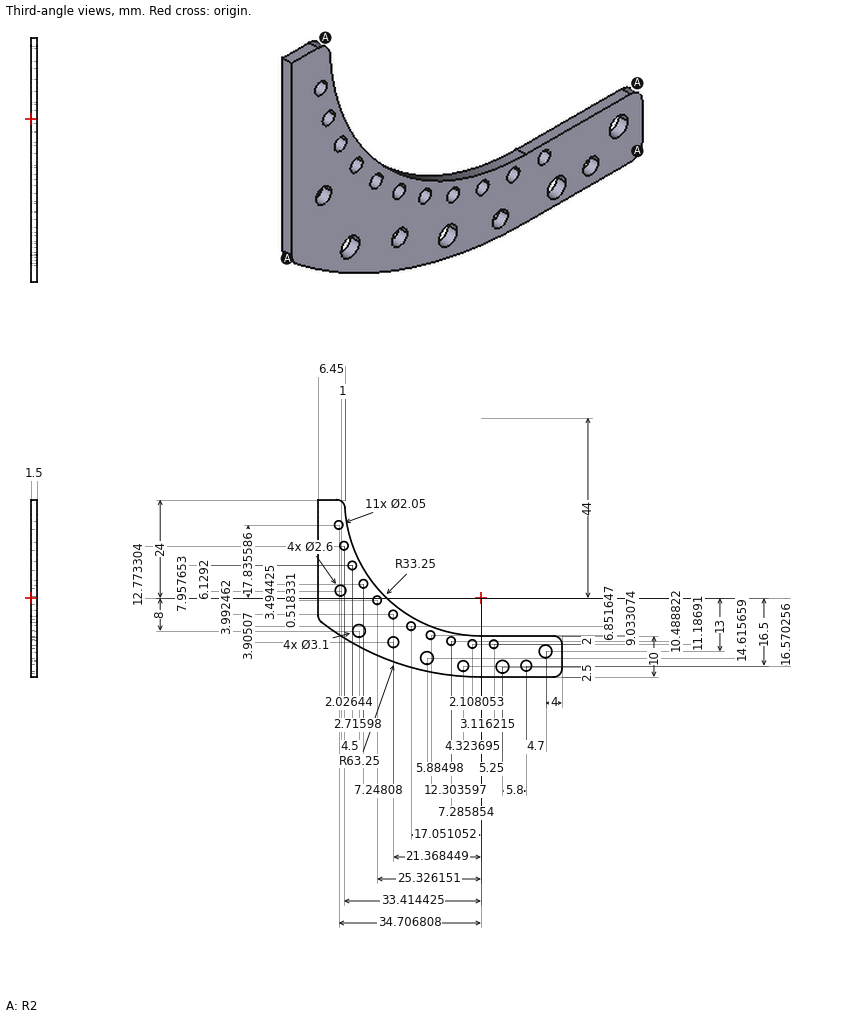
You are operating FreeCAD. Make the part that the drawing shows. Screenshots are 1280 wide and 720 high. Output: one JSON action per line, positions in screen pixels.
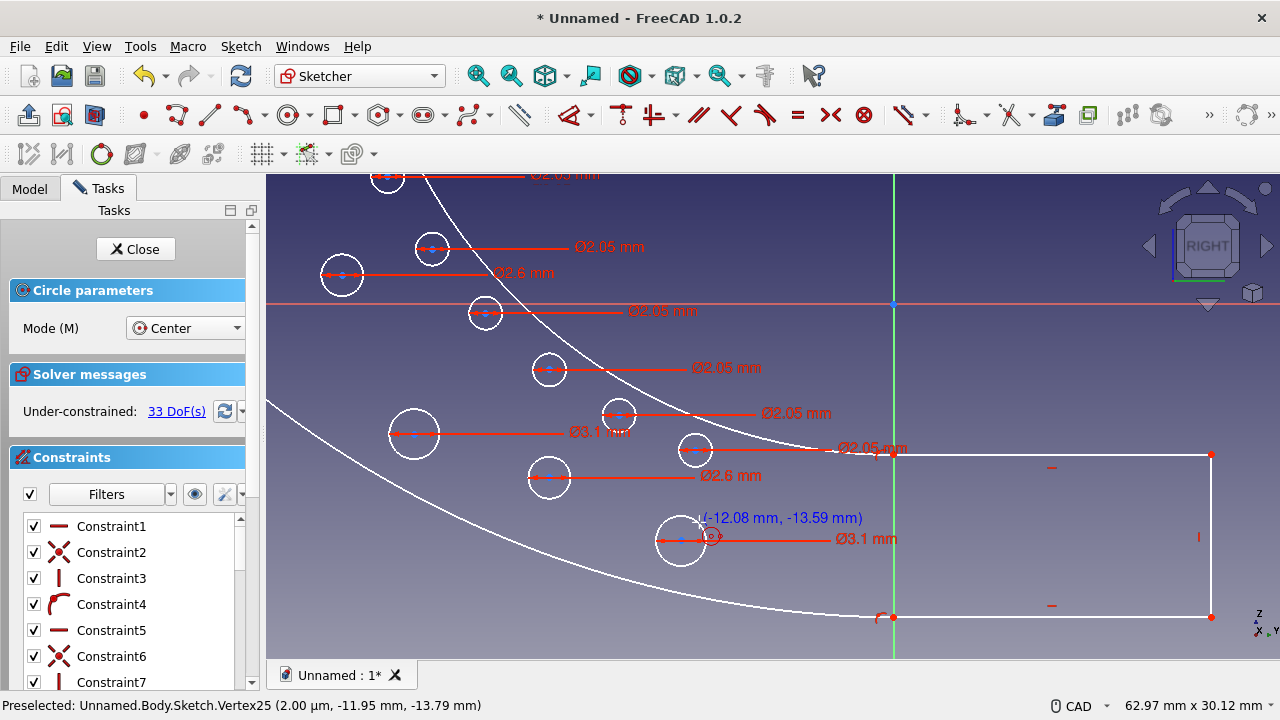
{"action": "scroll", "coordinate": [776, 473], "scroll_direction": "up", "scroll_amount": 2}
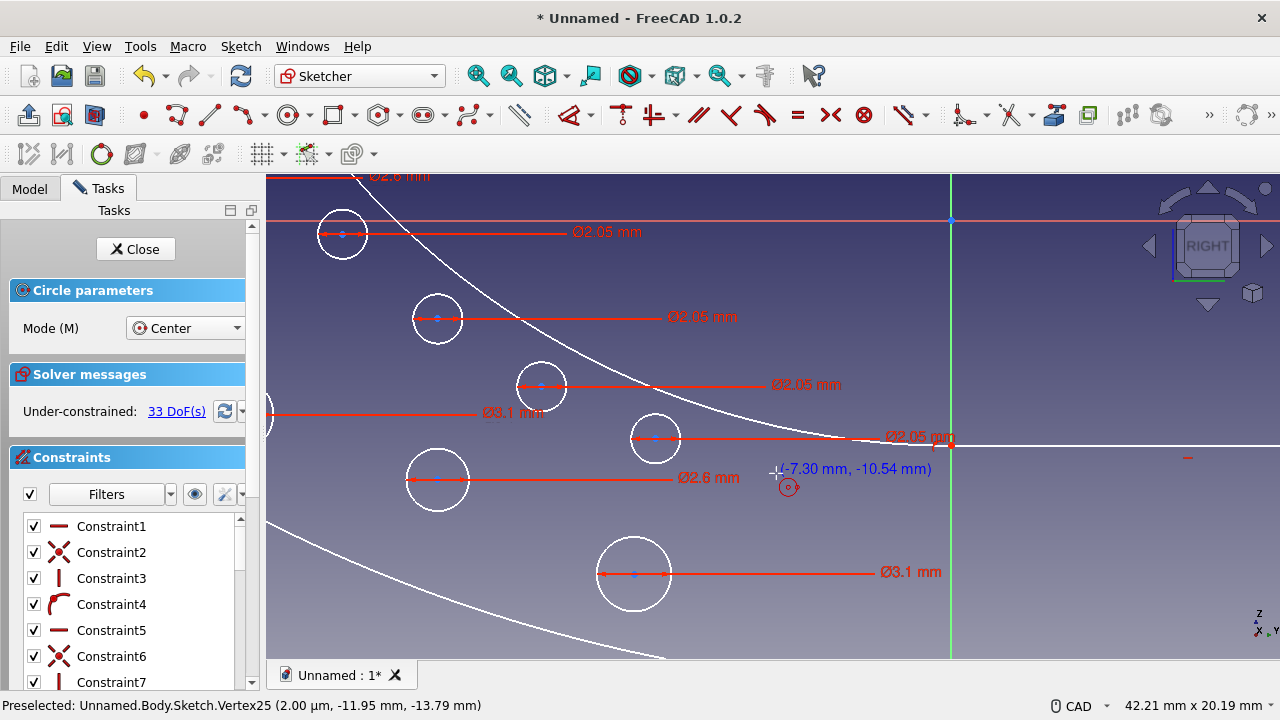
{"action": "left_click", "coordinate": [776, 473]}
{"action": "mouse_move", "coordinate": [794, 455]}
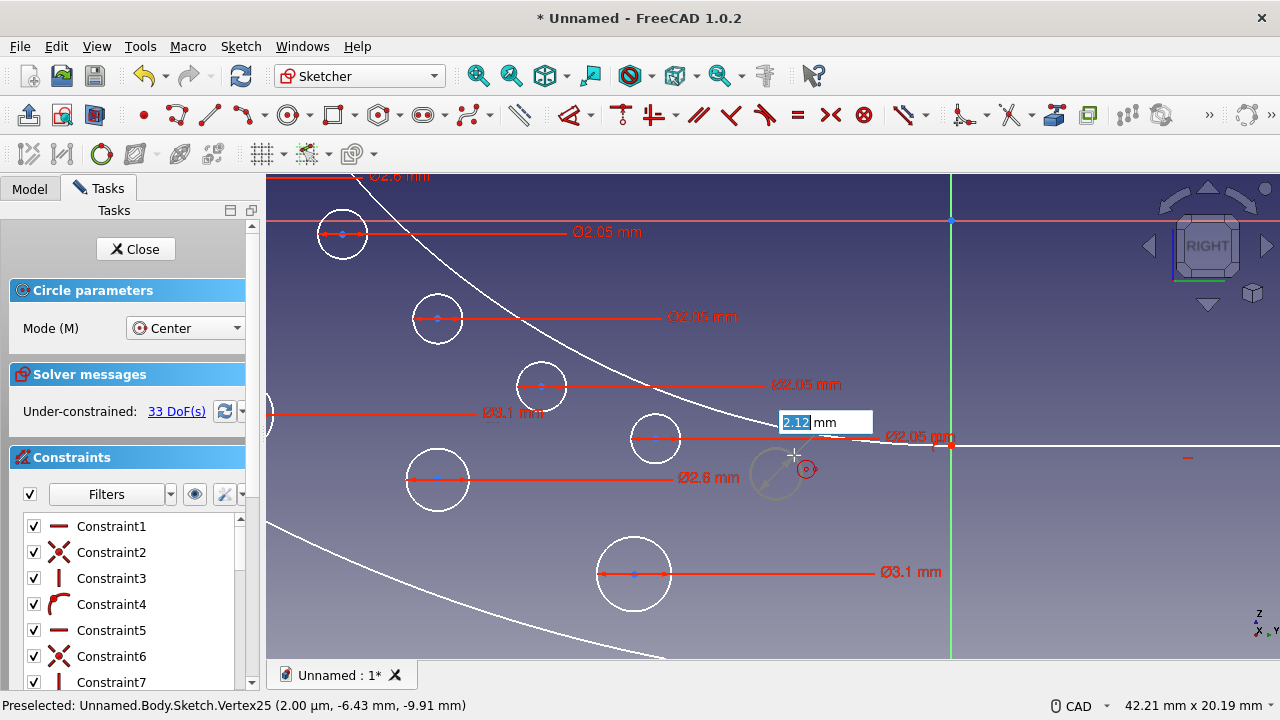
{"action": "type", "text": "2.05"}
{"action": "key", "text": "Return"}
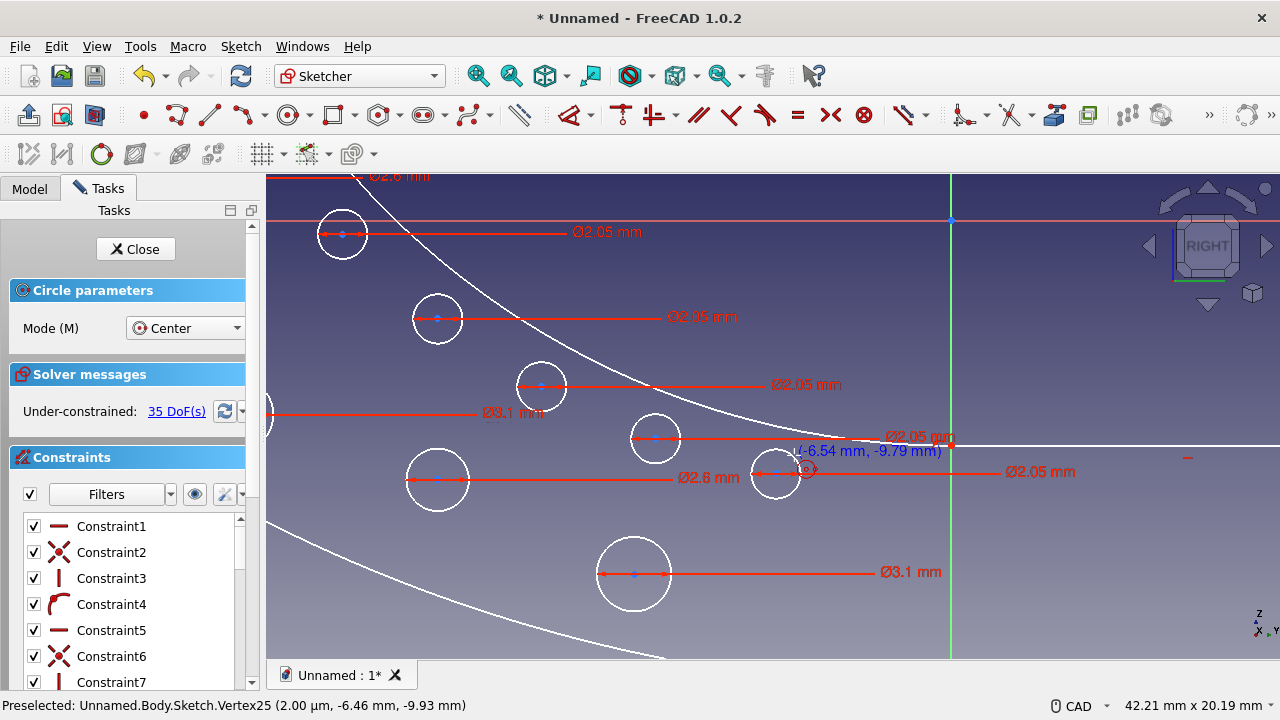
{"action": "left_click", "coordinate": [847, 619]}
{"action": "mouse_move", "coordinate": [869, 597]}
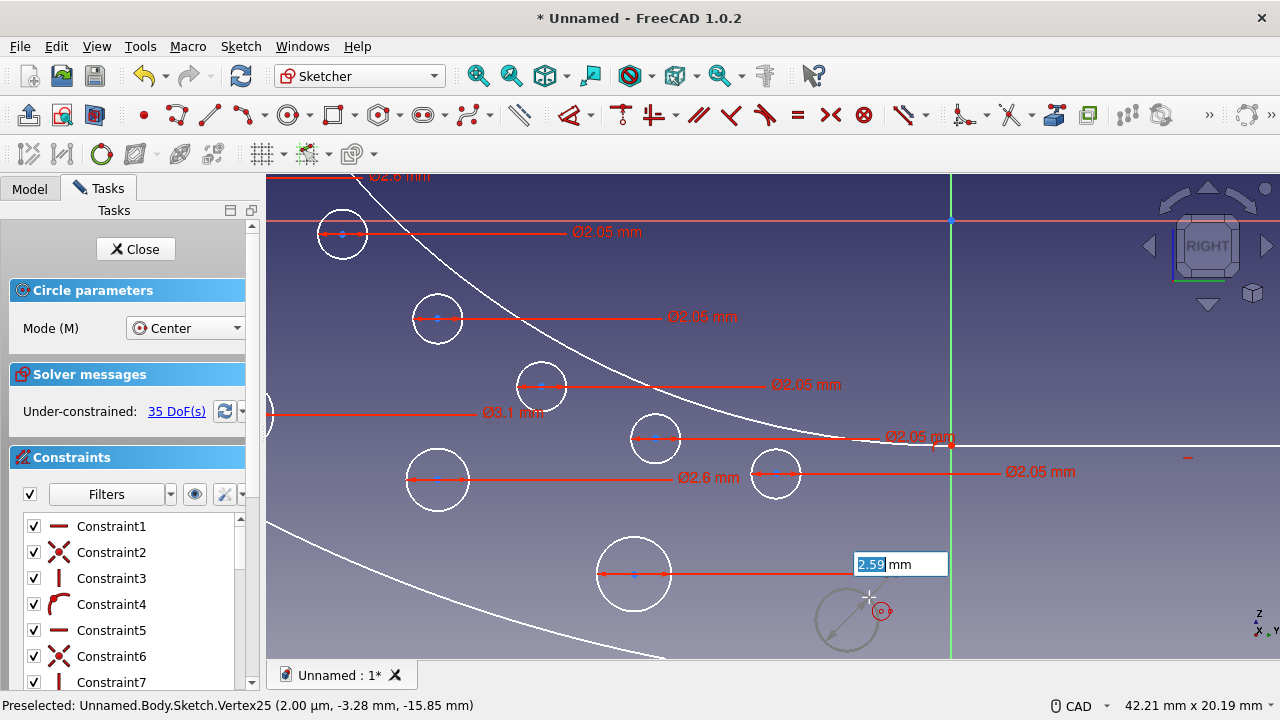
{"action": "type", "text": "2.6"}
{"action": "key", "text": "Return"}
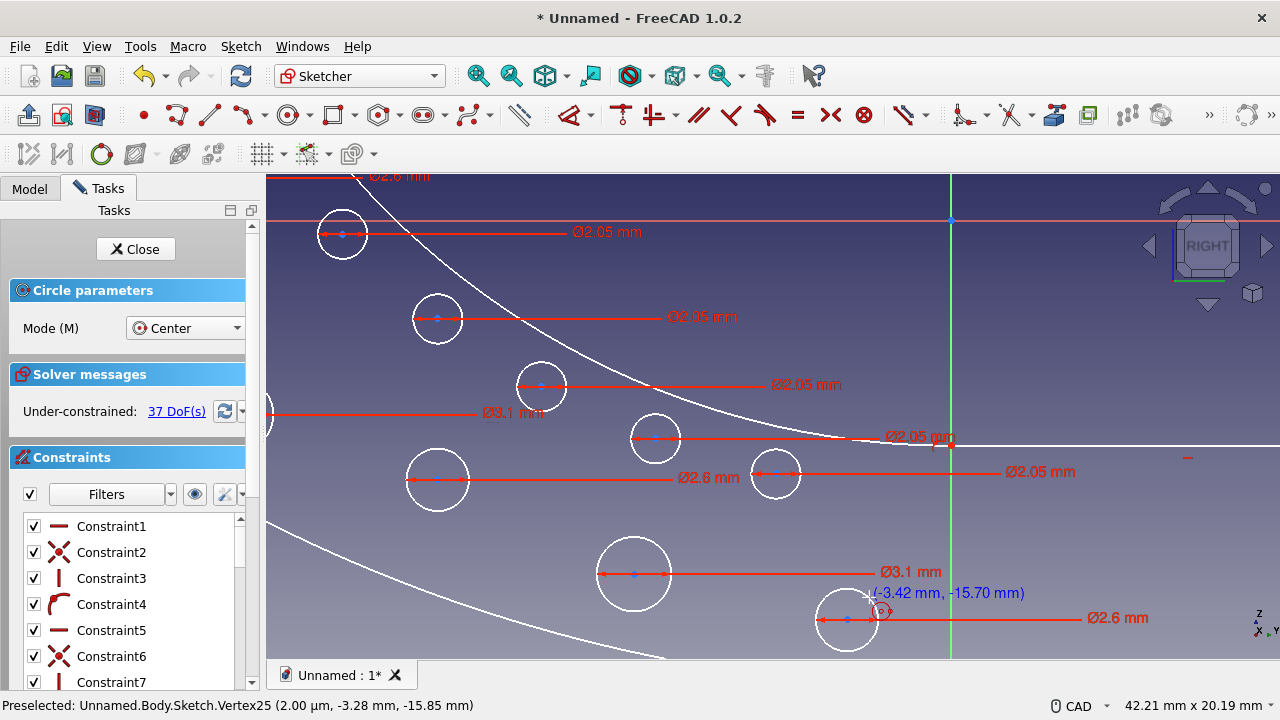
{"action": "left_click", "coordinate": [900, 490]}
{"action": "mouse_move", "coordinate": [918, 472]}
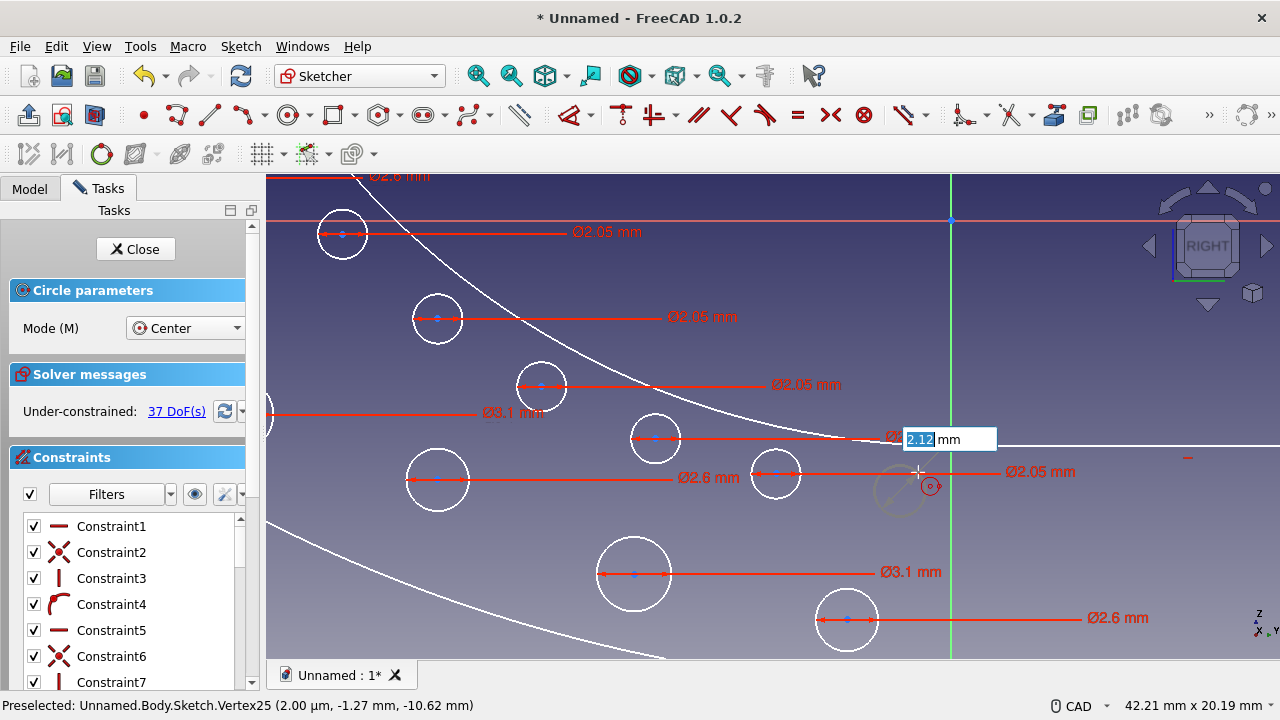
{"action": "type", "text": "2.05"}
{"action": "key", "text": "Return"}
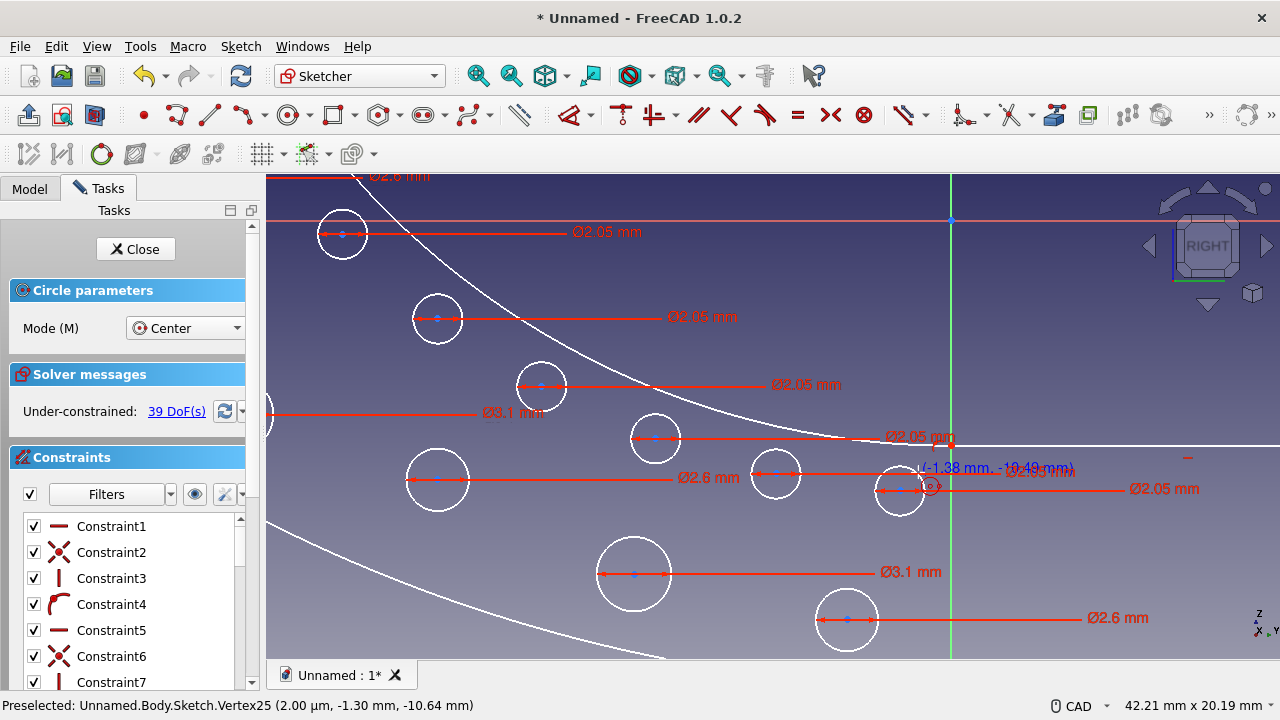
{"action": "left_click", "coordinate": [1026, 491]}
{"action": "mouse_move", "coordinate": [1043, 474]}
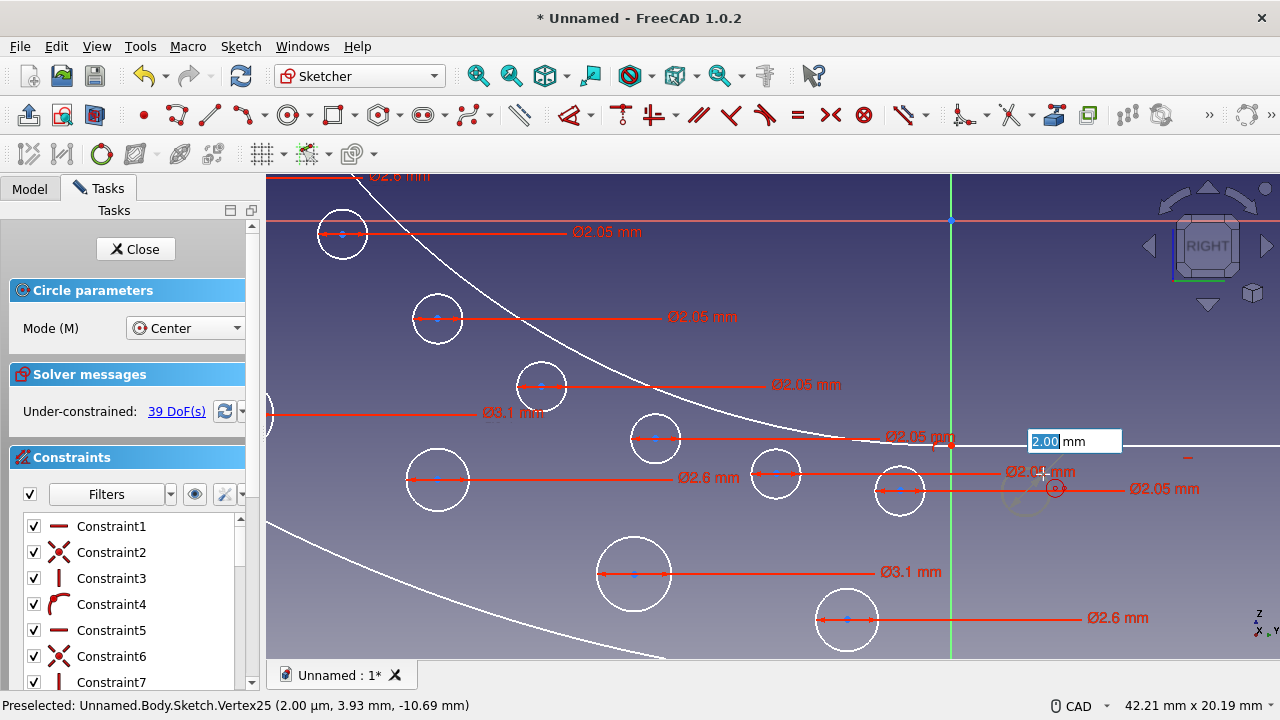
{"action": "type", "text": "2.05"}
{"action": "key", "text": "Return"}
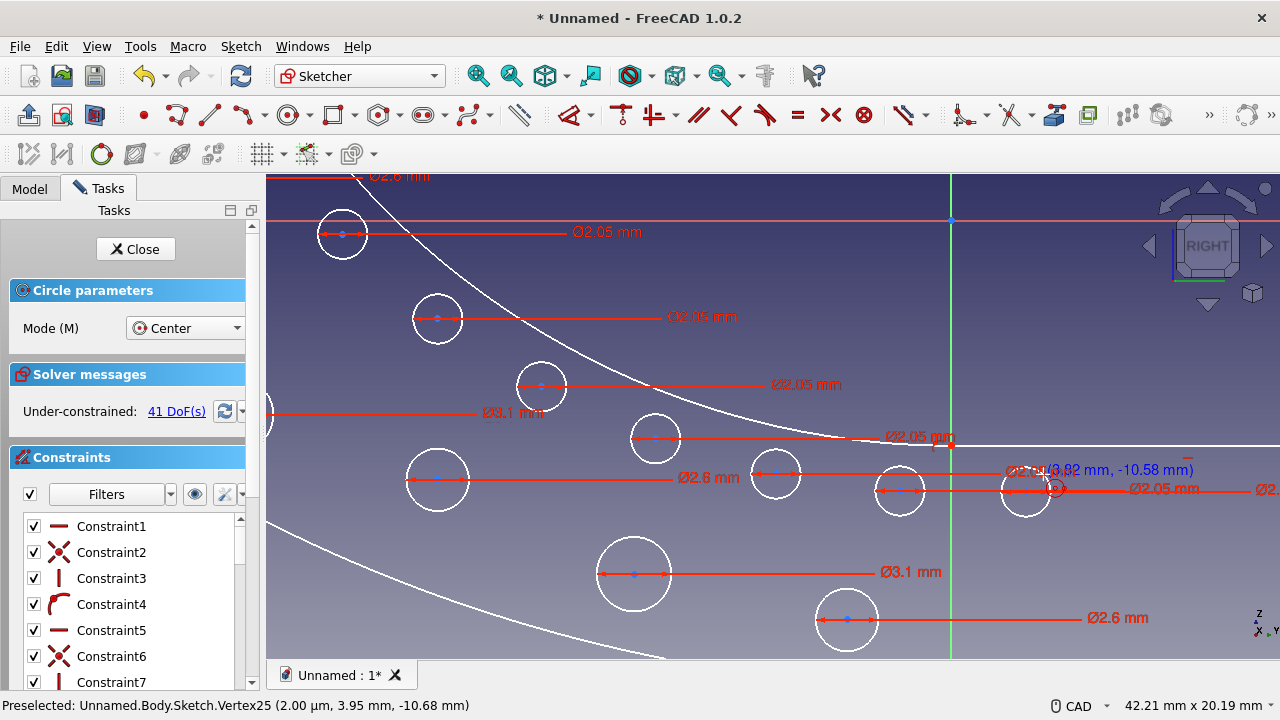
{"action": "left_click", "coordinate": [1077, 623]}
{"action": "mouse_move", "coordinate": [1104, 597]}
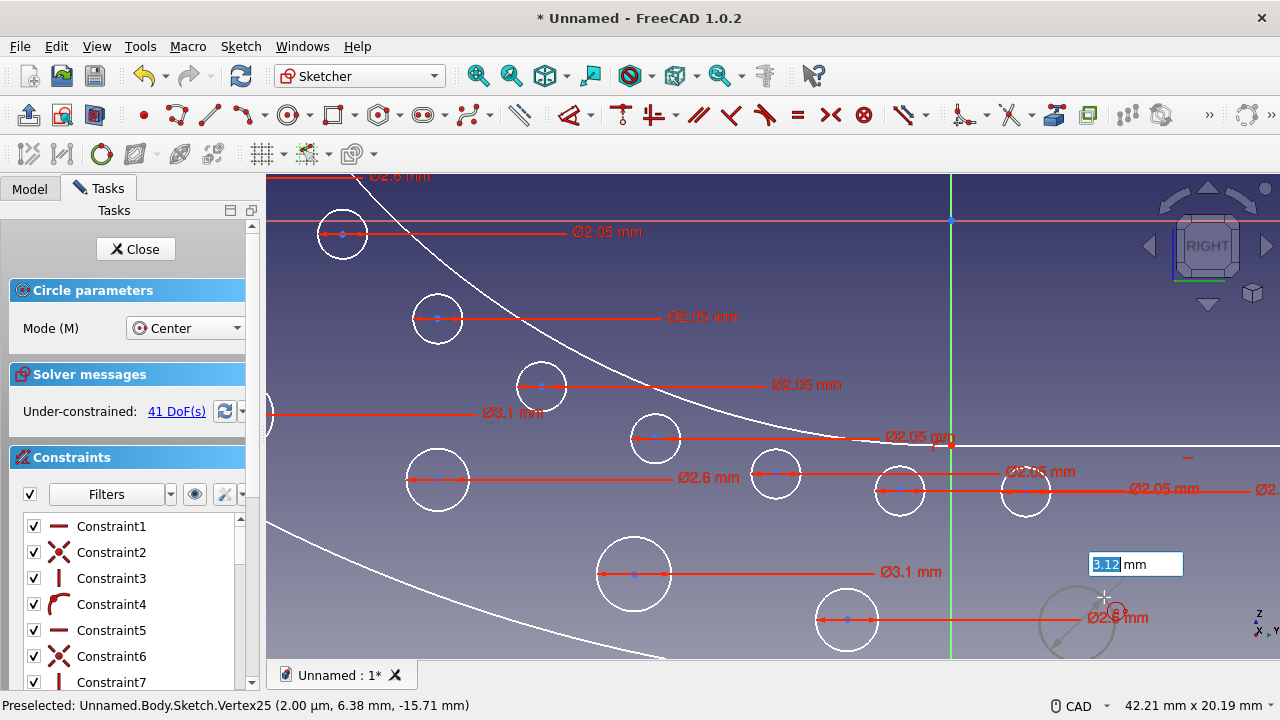
{"action": "type", "text": "3.1"}
{"action": "key", "text": "Return"}